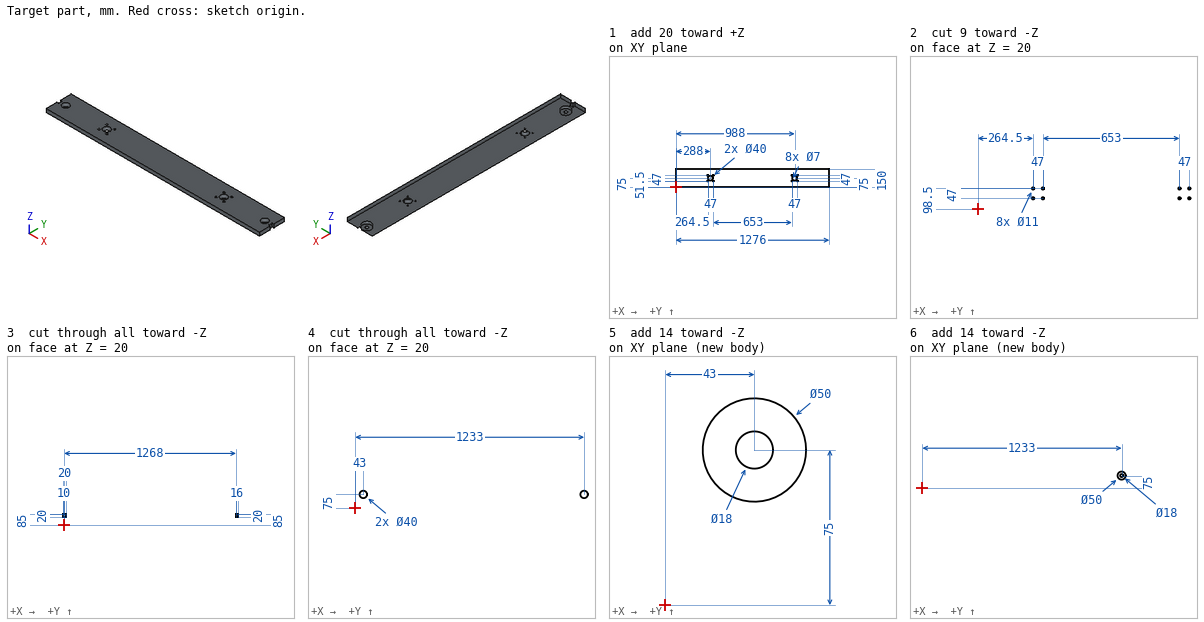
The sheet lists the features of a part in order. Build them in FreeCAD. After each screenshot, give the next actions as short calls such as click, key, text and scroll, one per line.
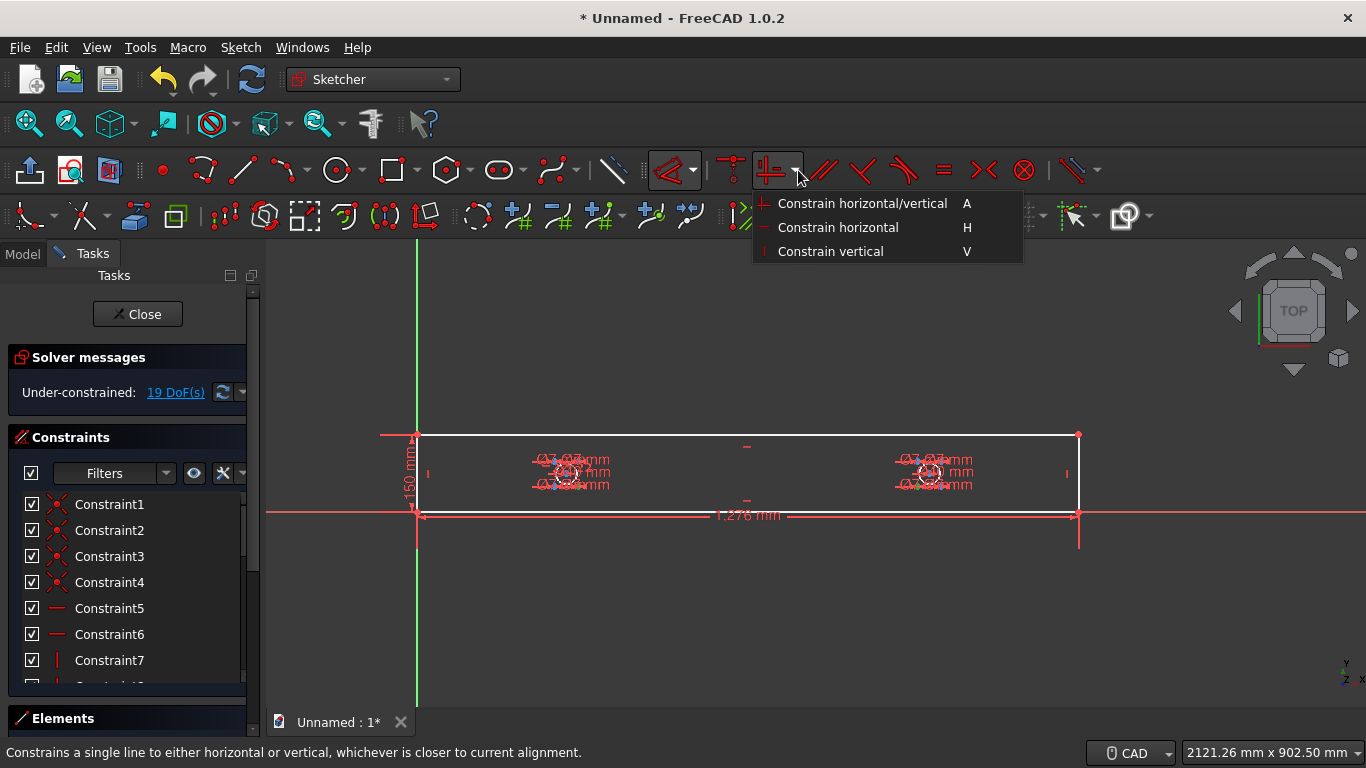
click(888, 227)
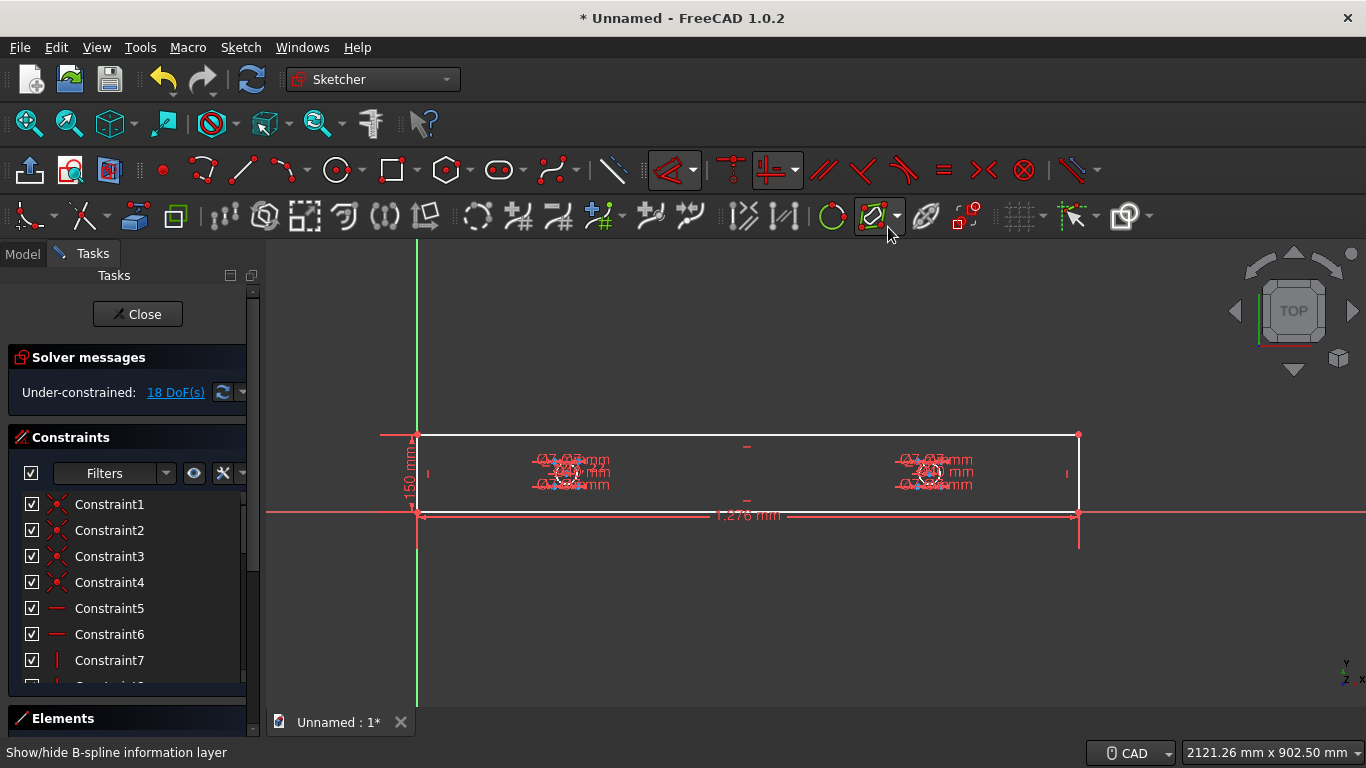
click(917, 487)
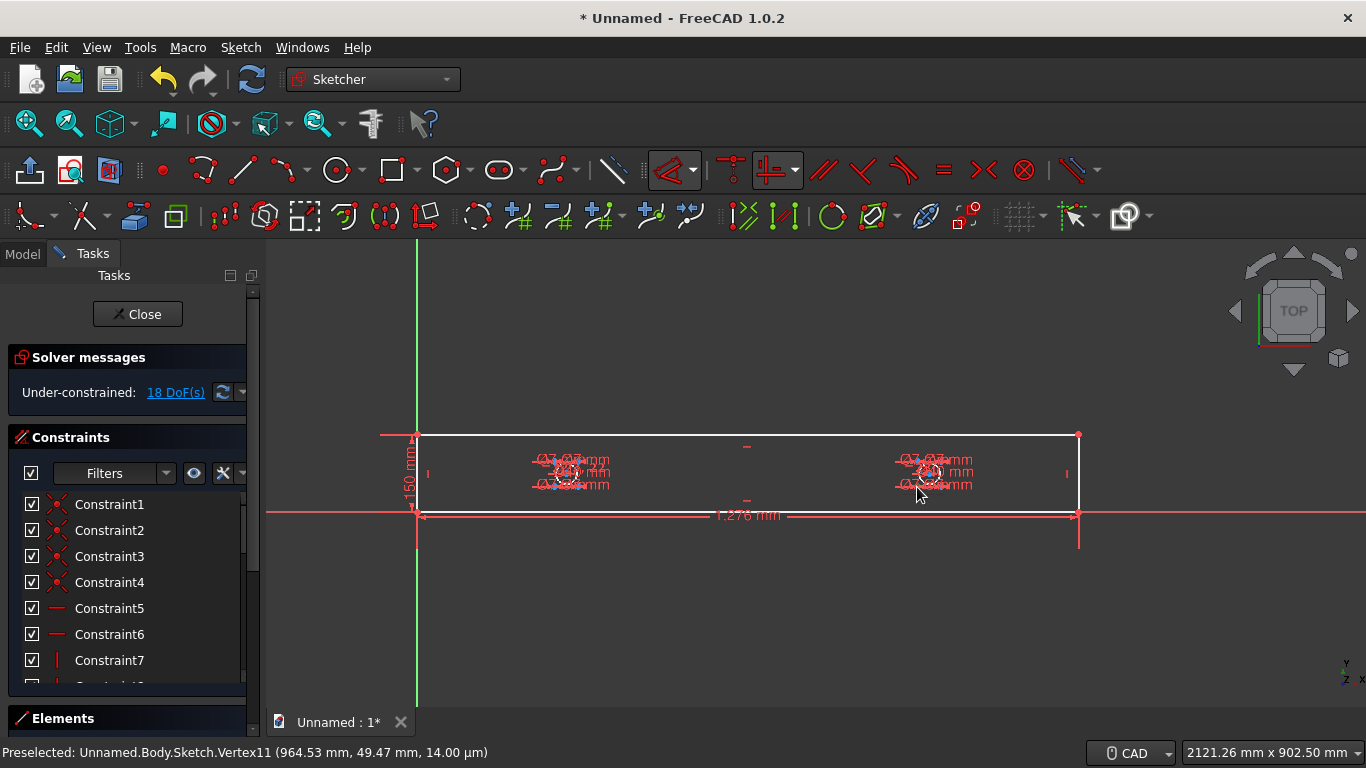
click(941, 487)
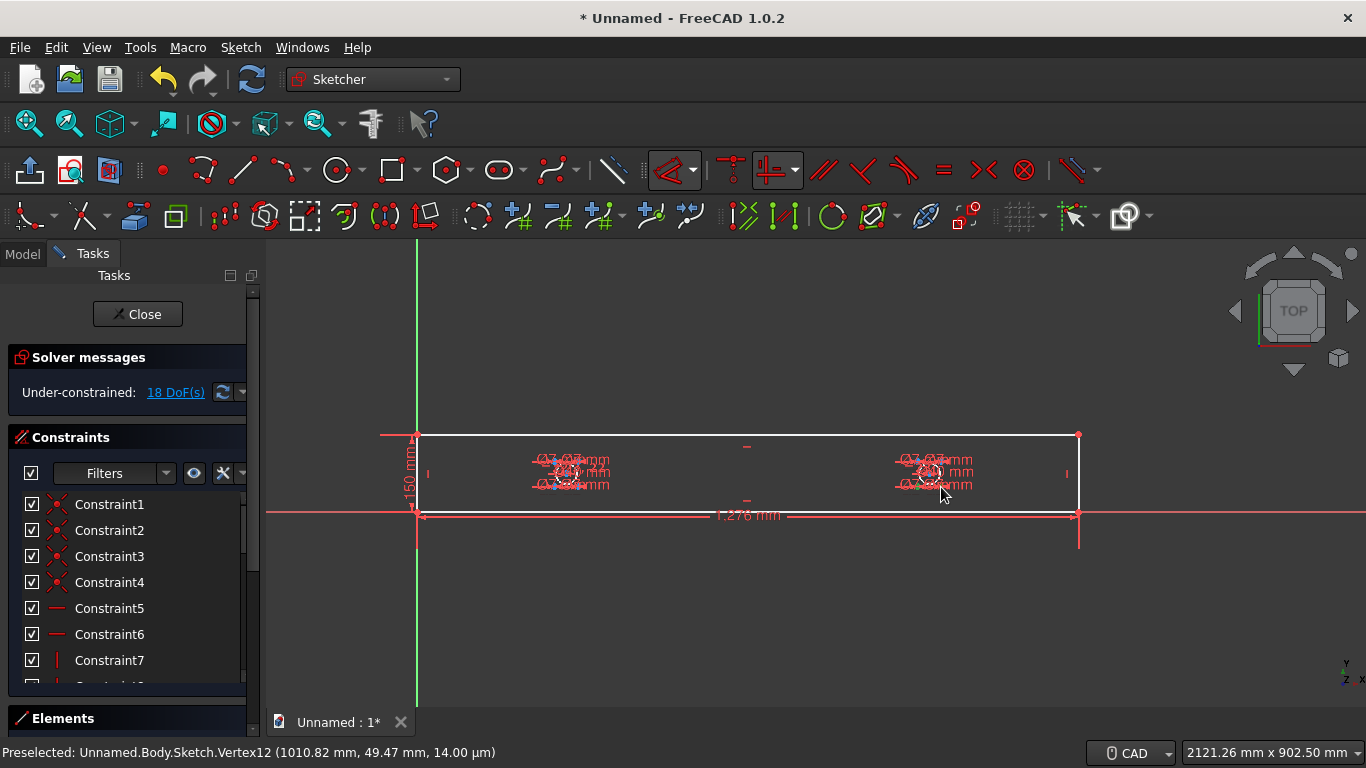
click(798, 170)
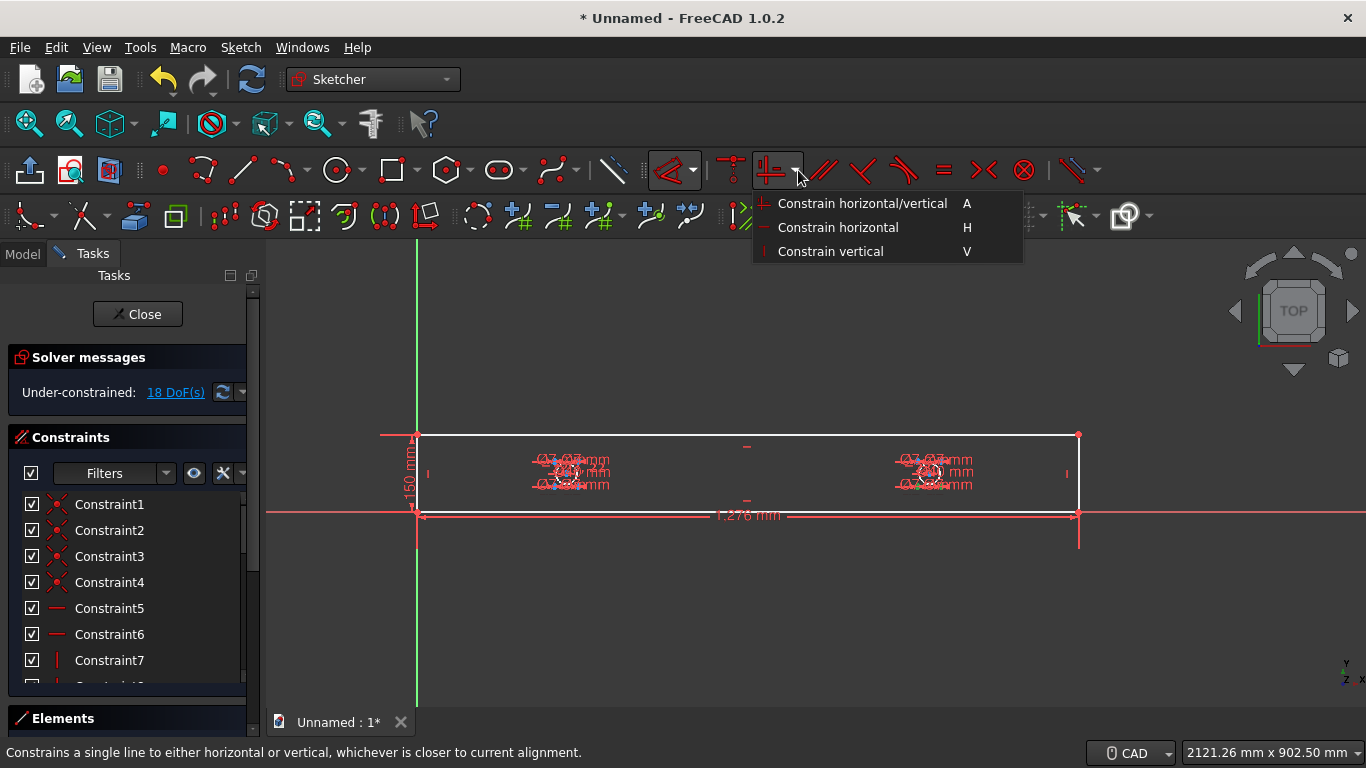
click(888, 227)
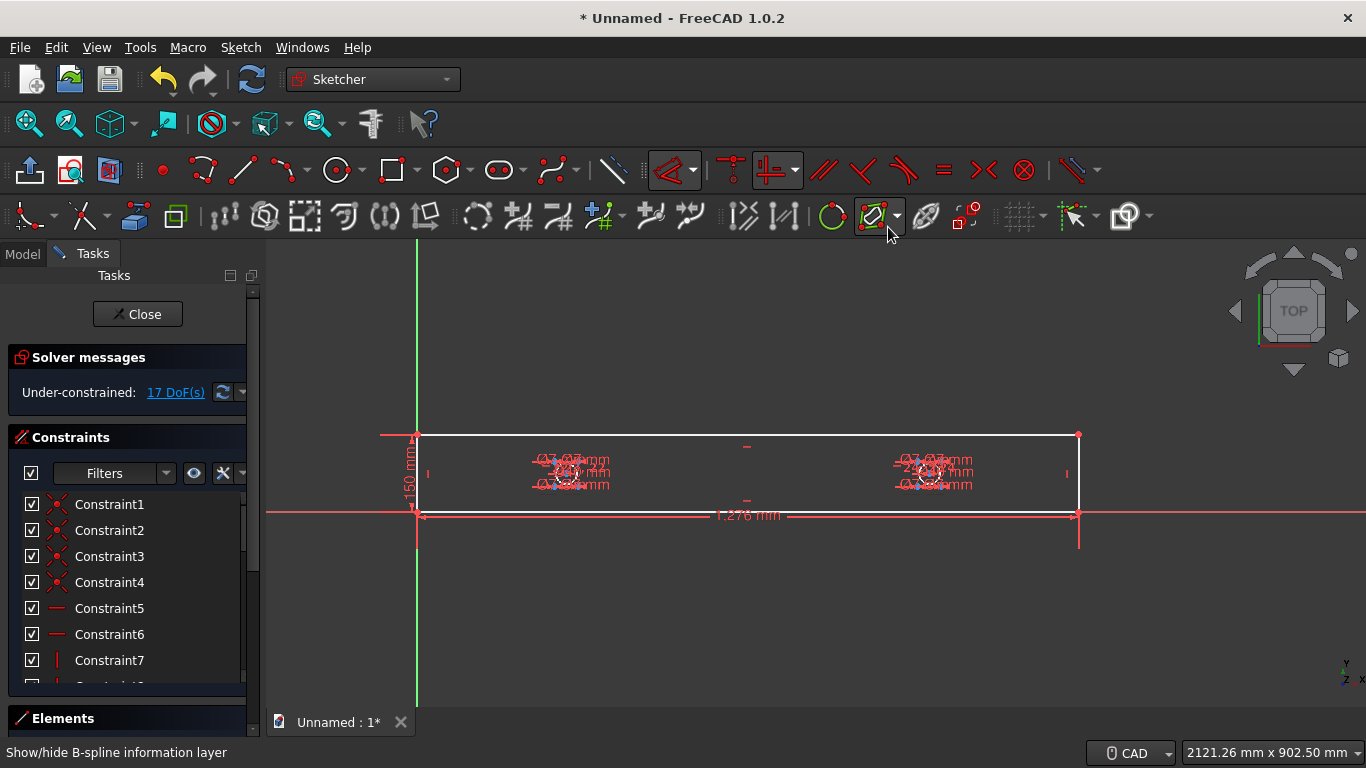
click(554, 487)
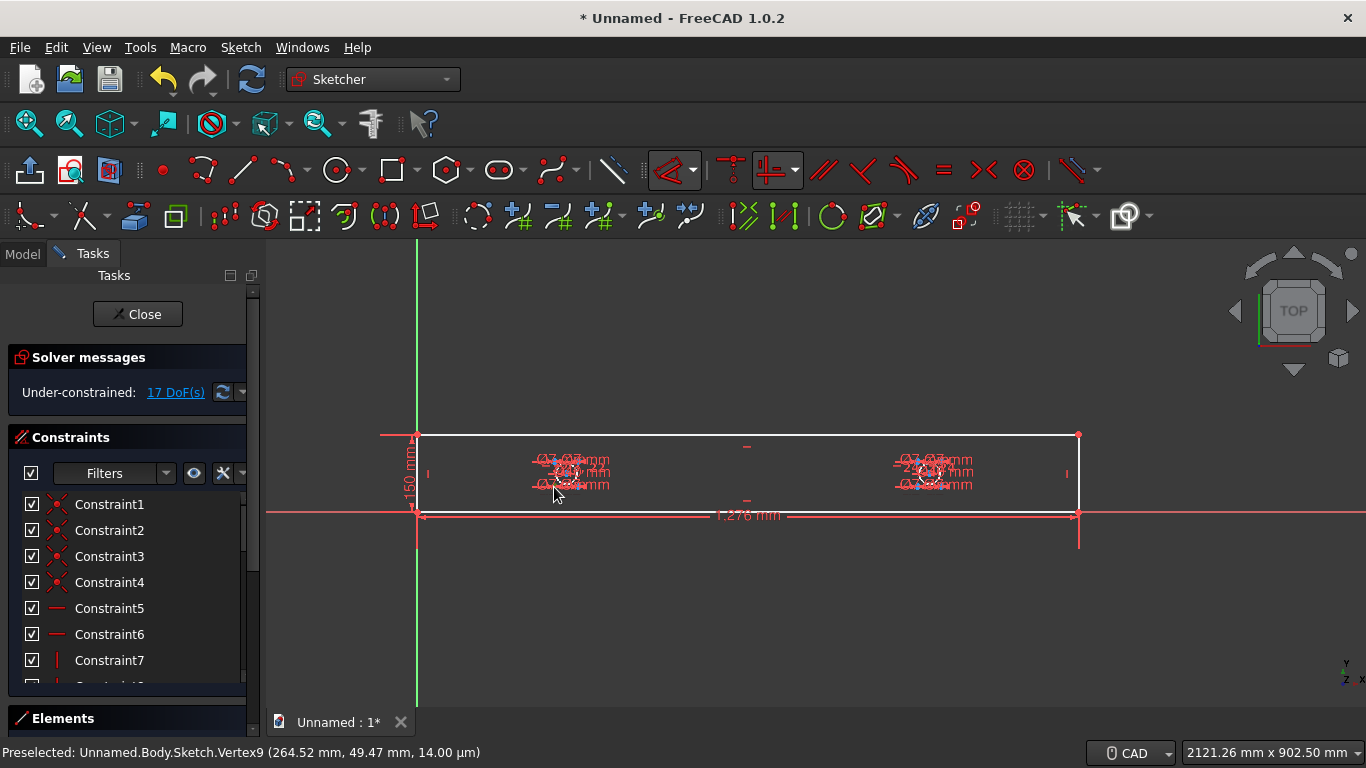
click(554, 462)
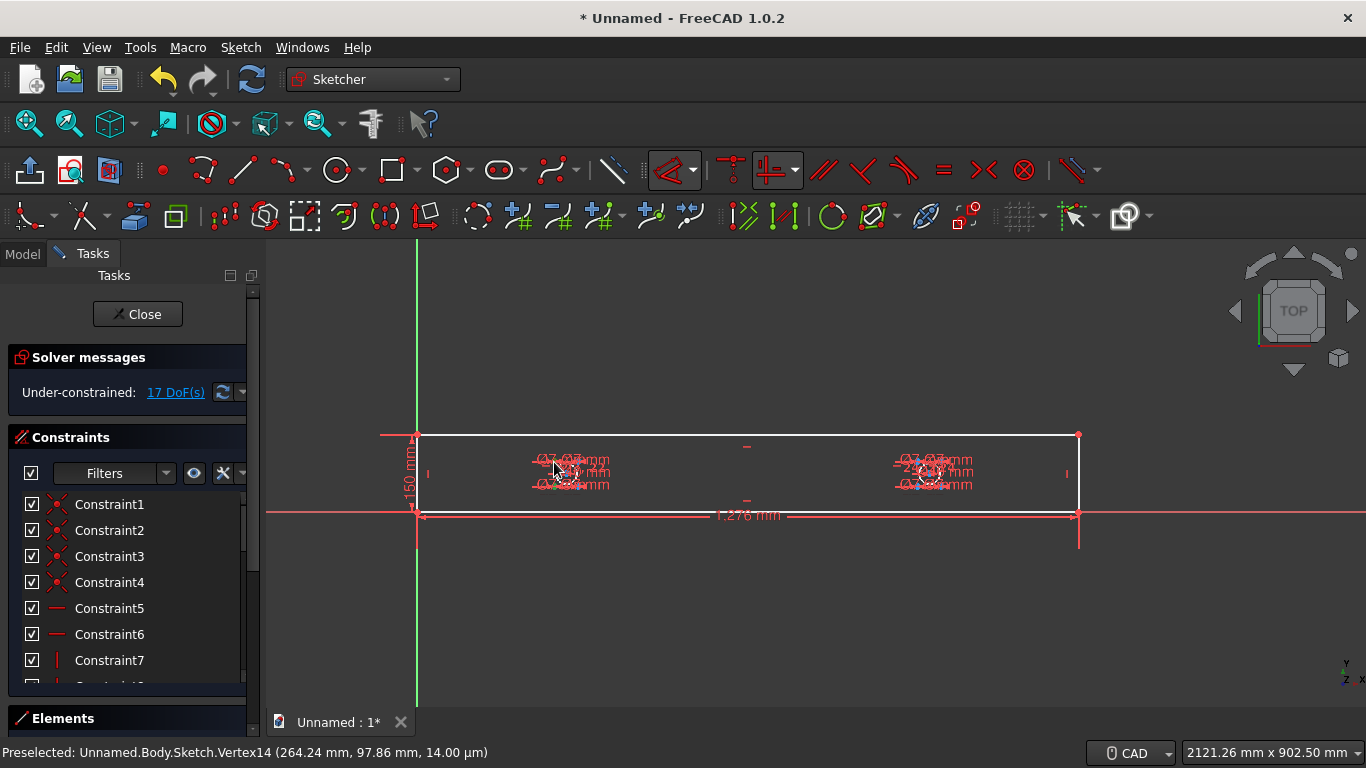
click(798, 170)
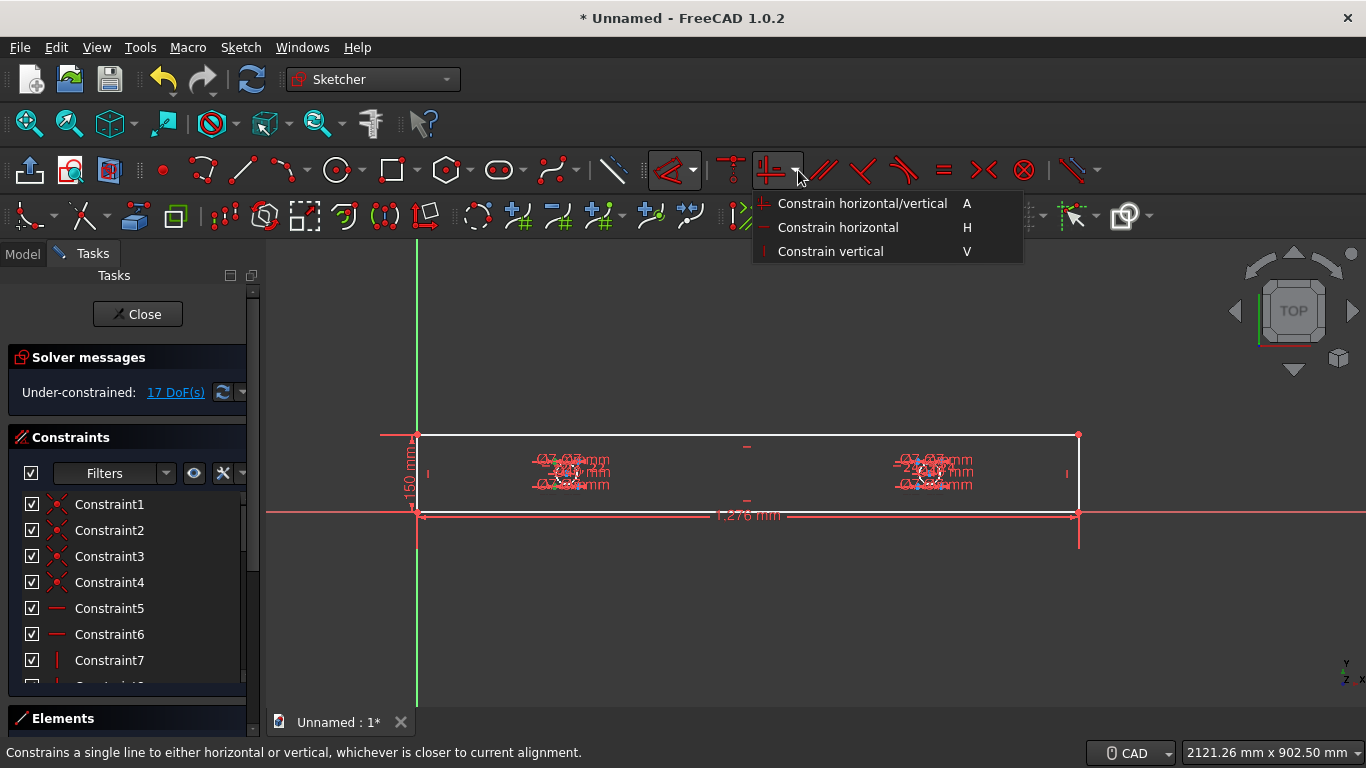
click(888, 251)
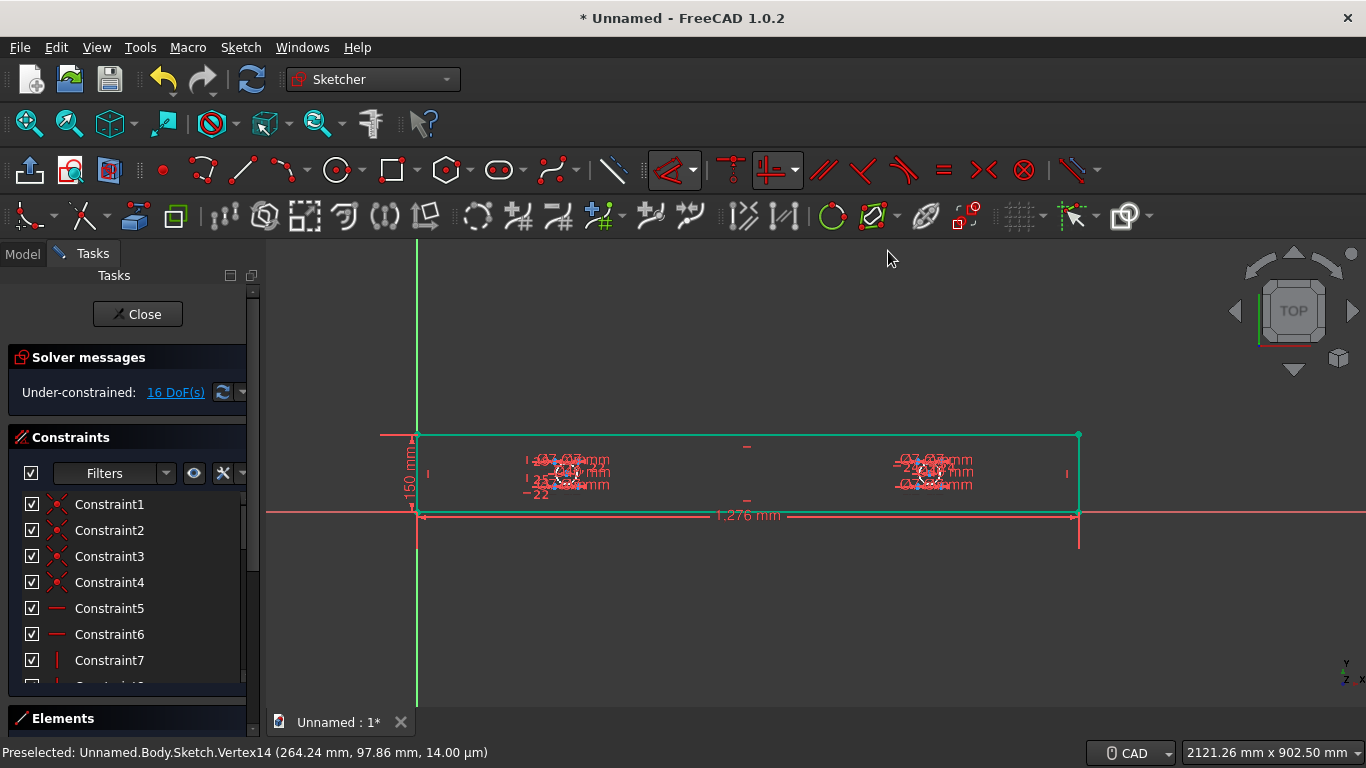
click(578, 487)